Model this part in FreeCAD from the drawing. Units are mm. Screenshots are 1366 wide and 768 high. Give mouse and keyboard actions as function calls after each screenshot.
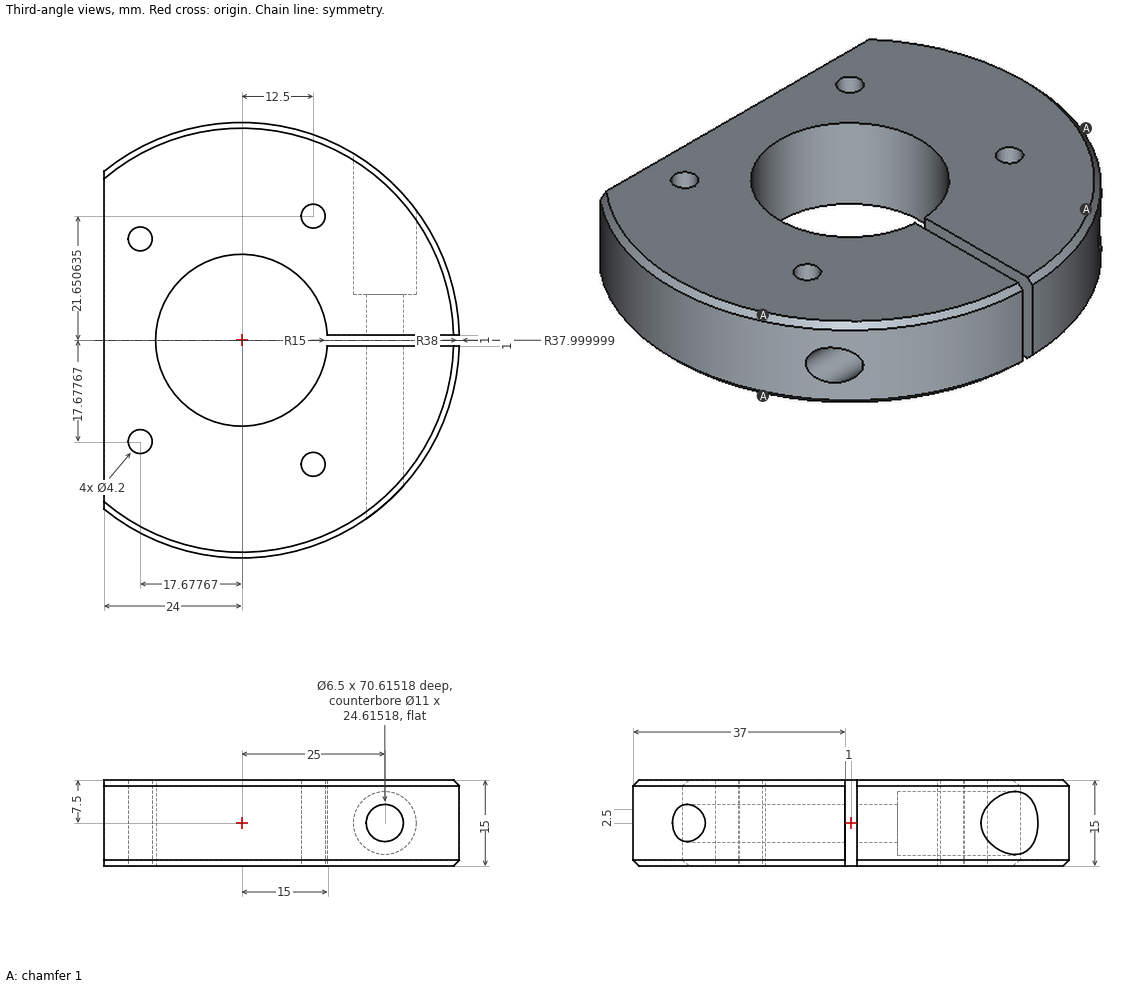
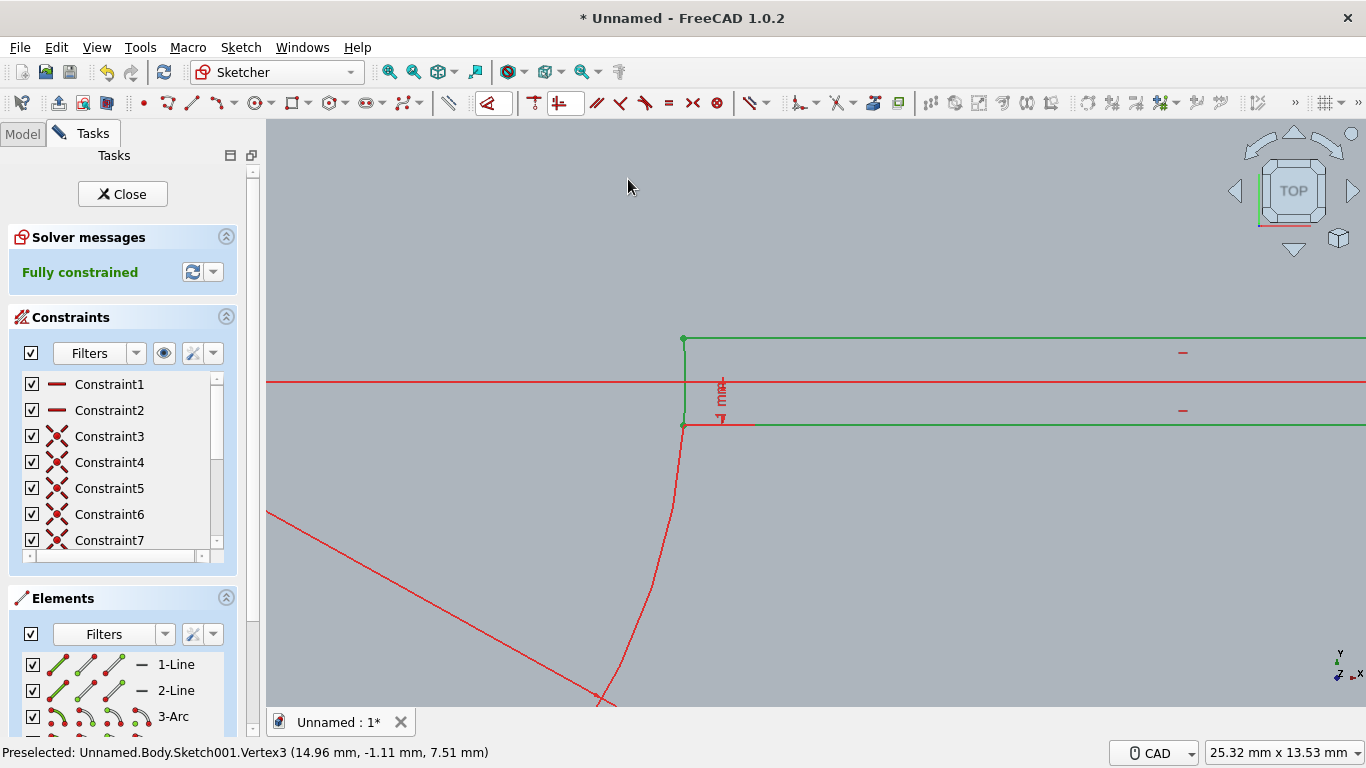
click(123, 194)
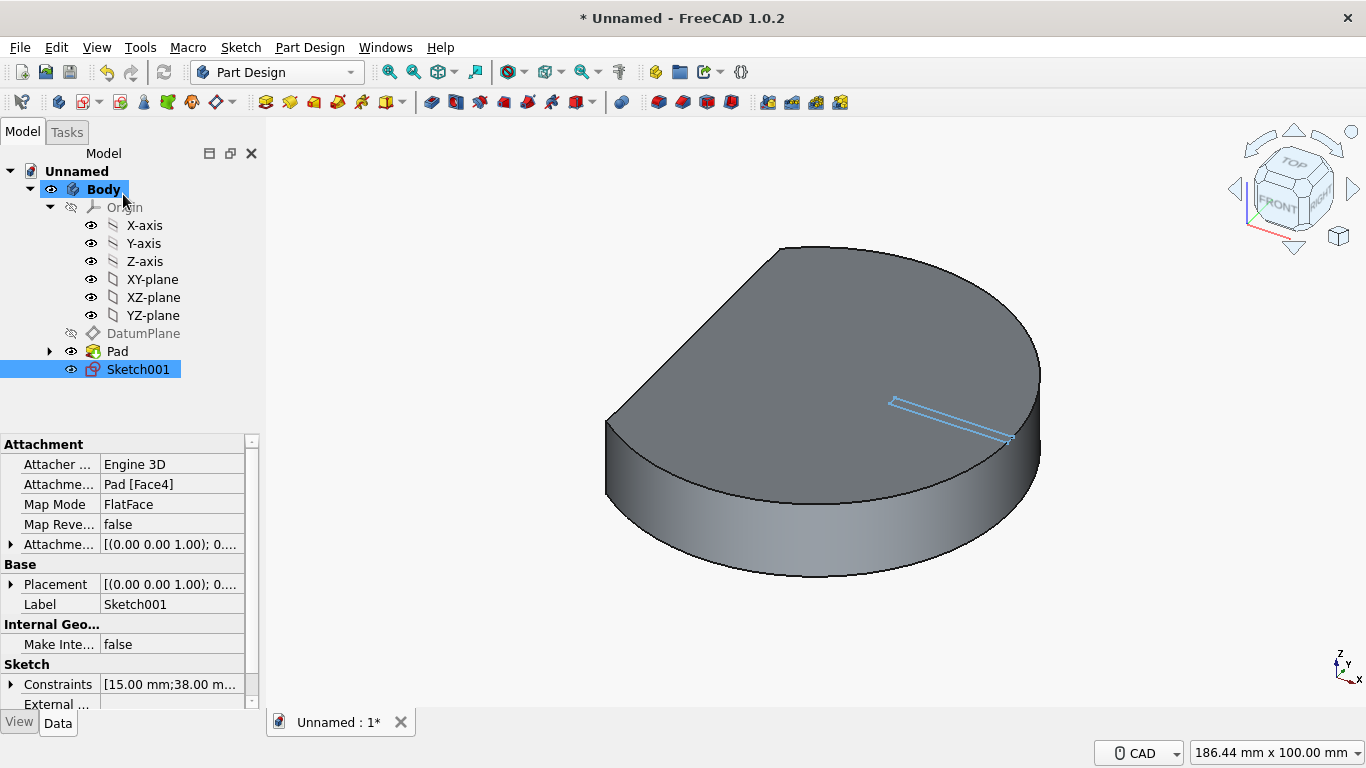
click(432, 102)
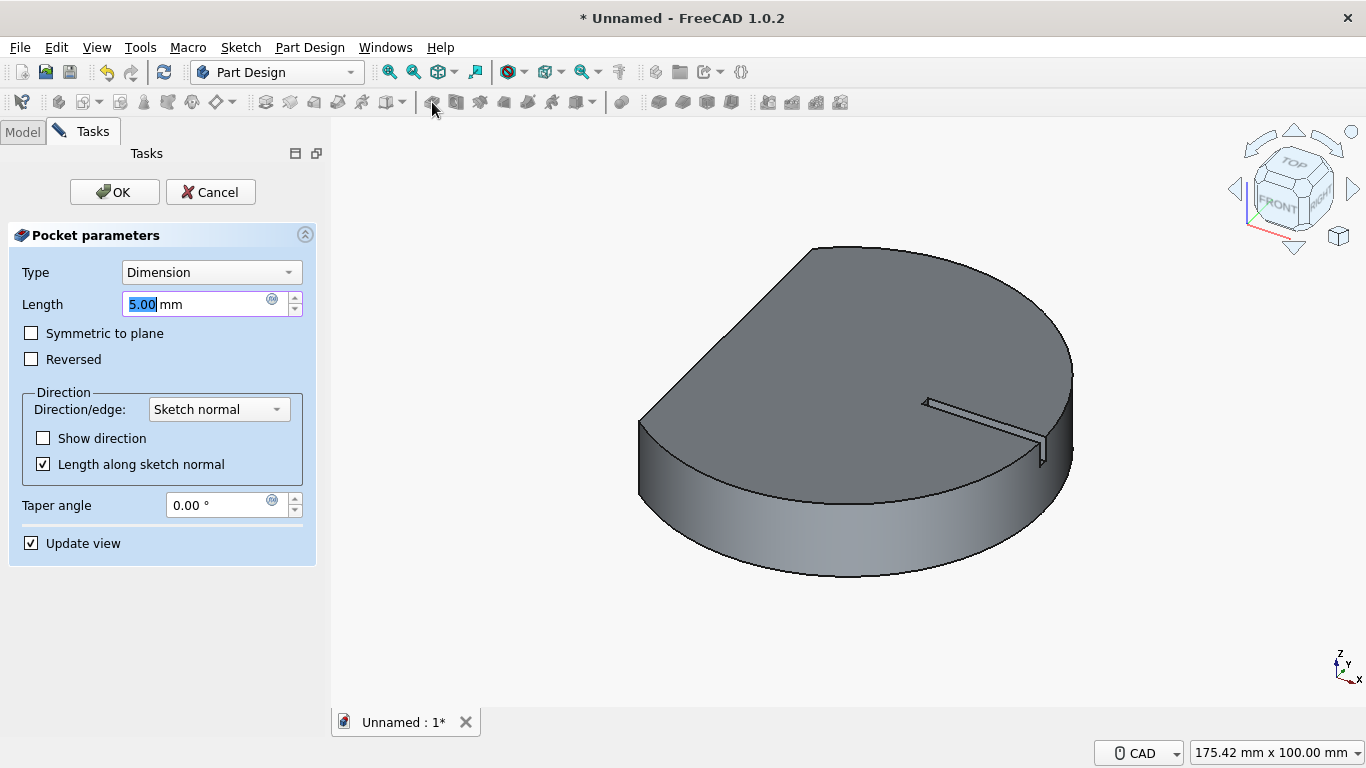
click(212, 272)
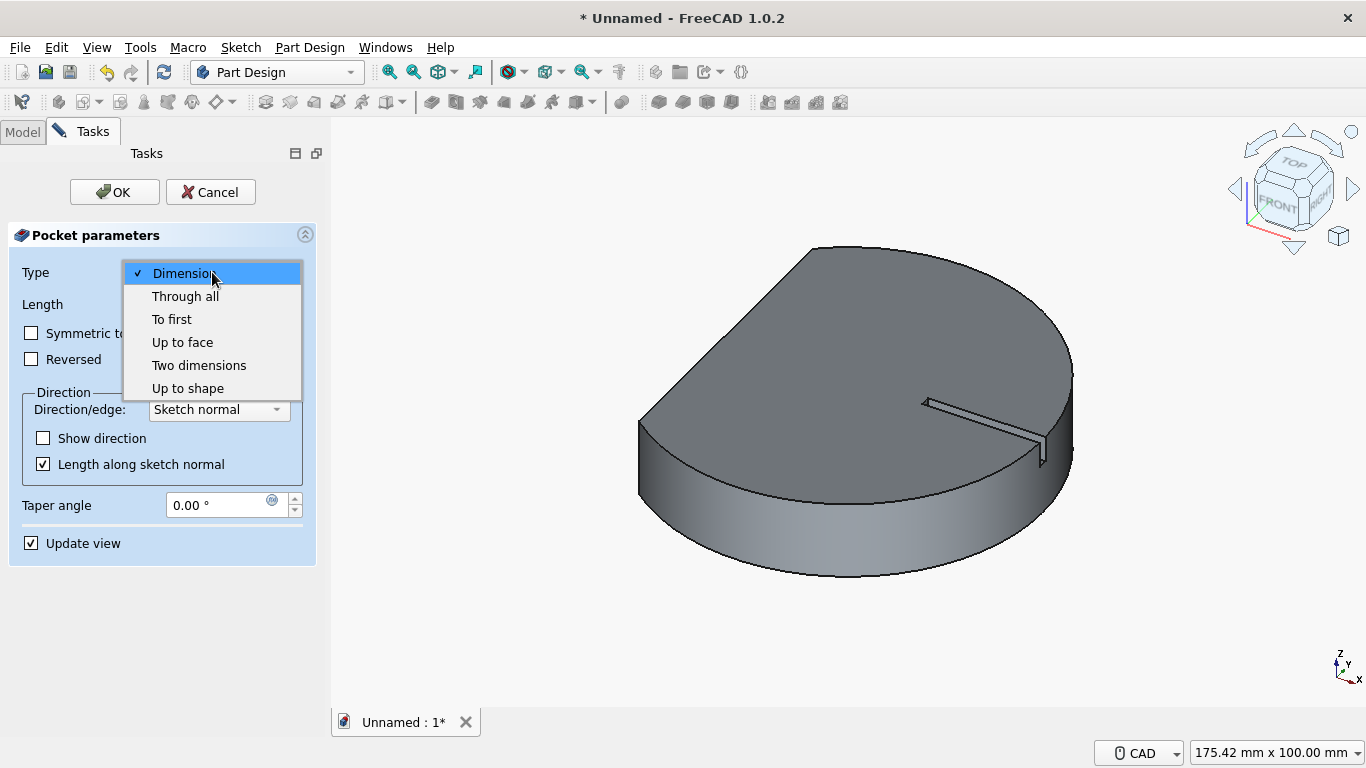
click(212, 296)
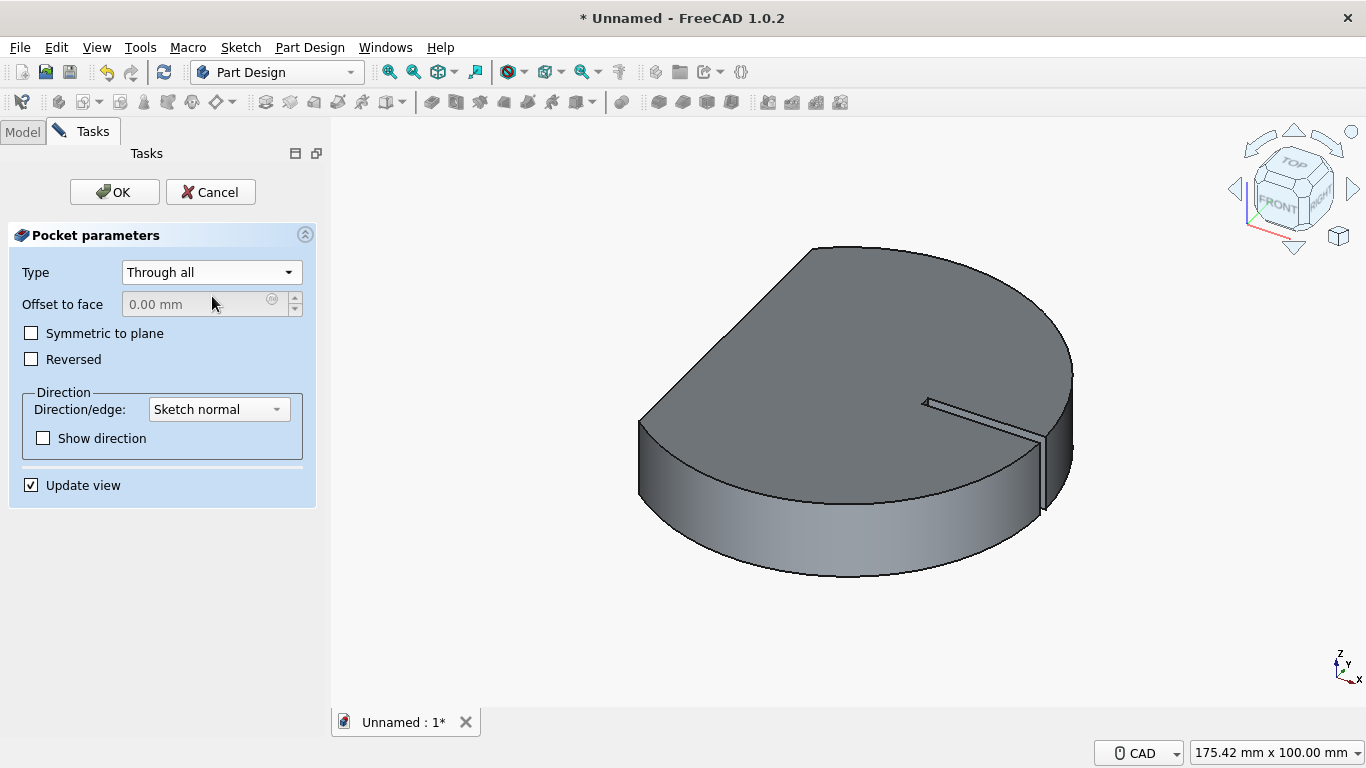
click(115, 192)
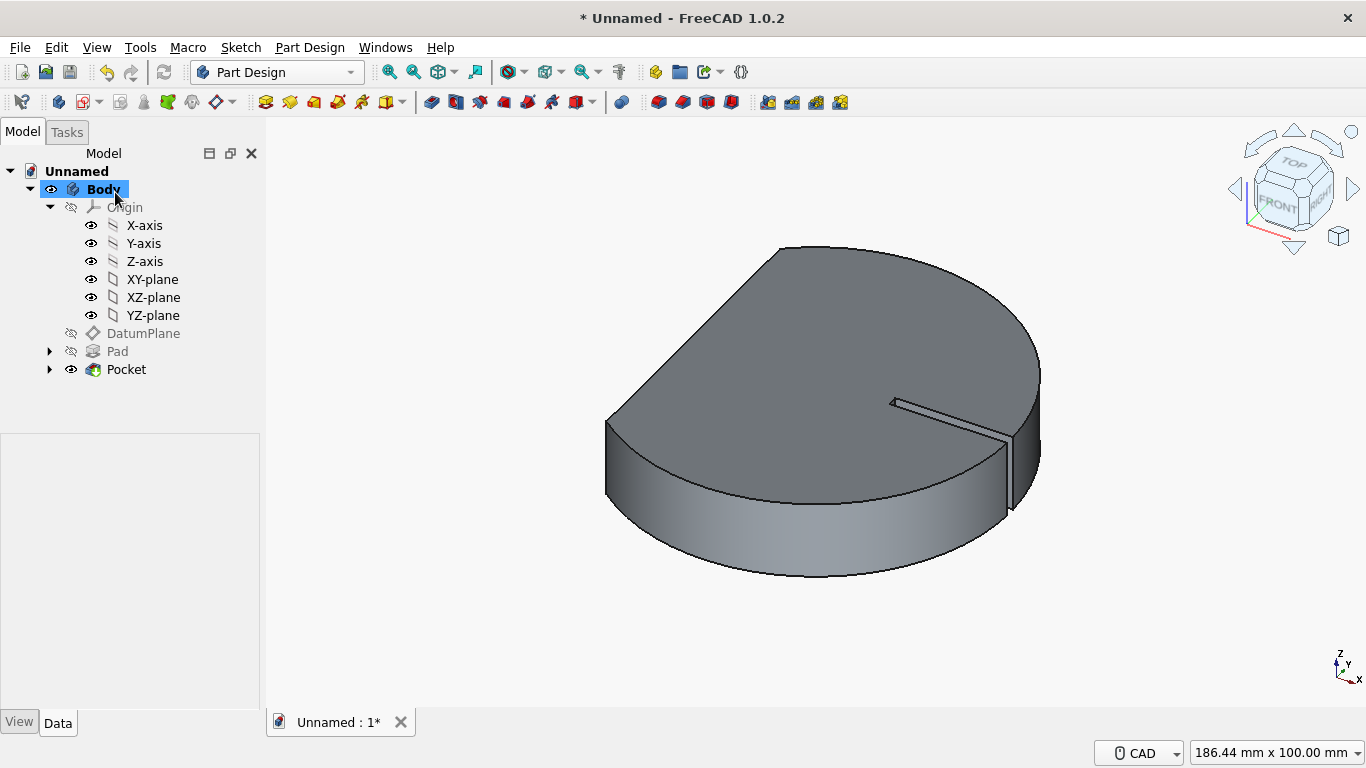
click(84, 102)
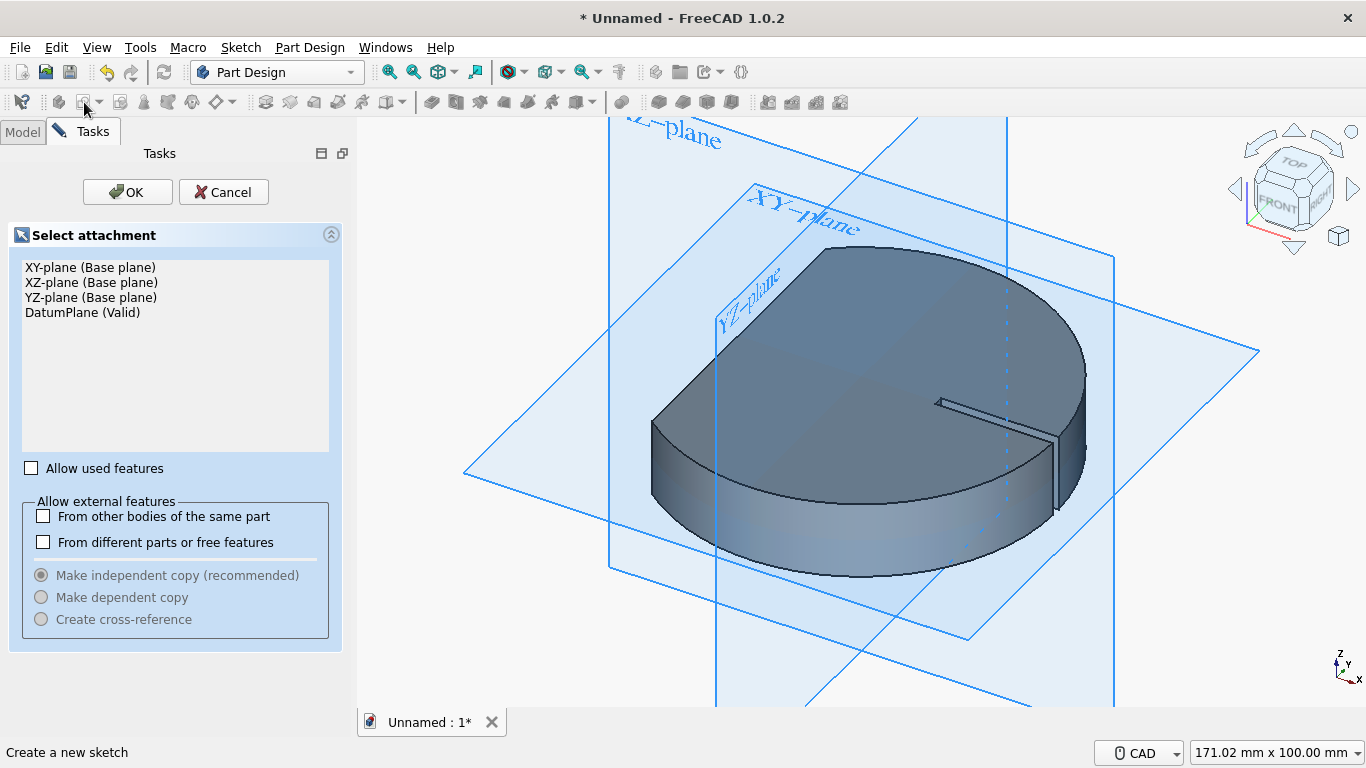
click(82, 282)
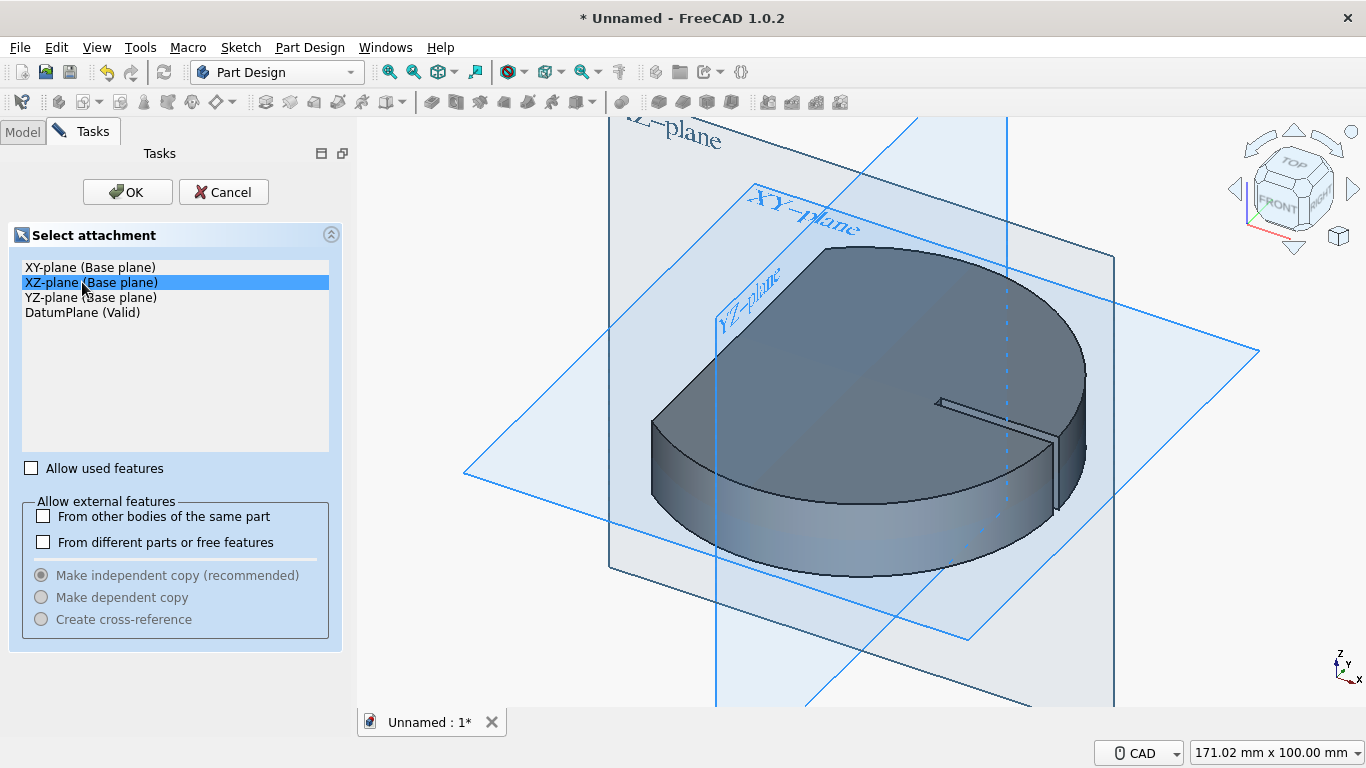
click(128, 192)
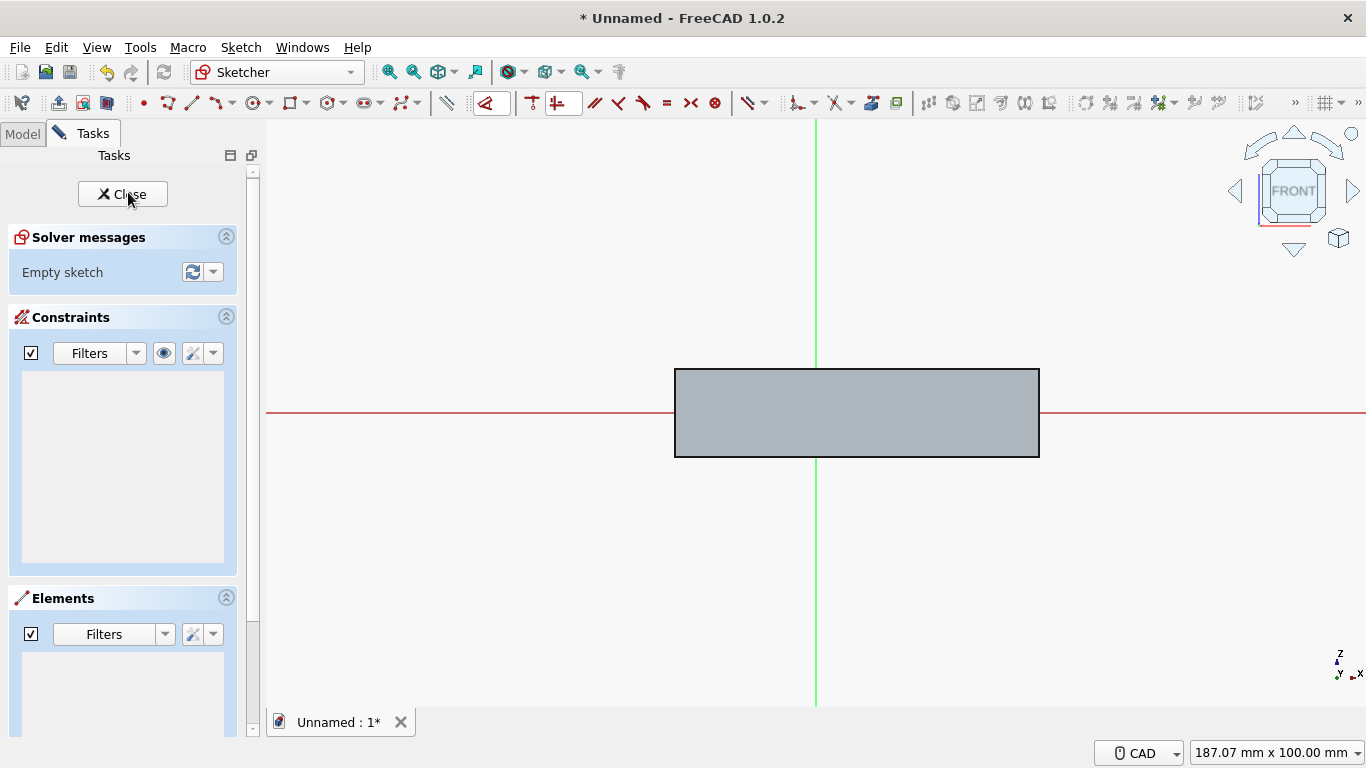
click(108, 104)